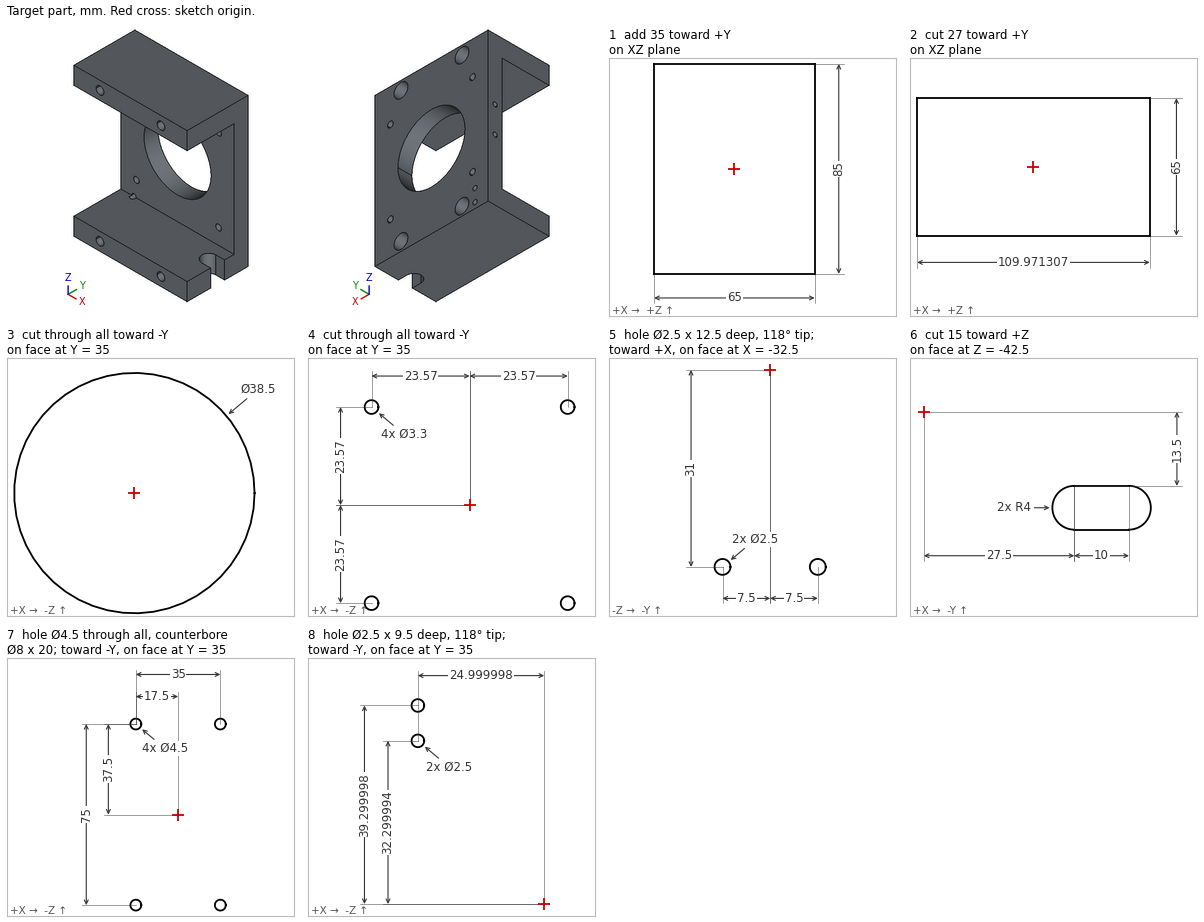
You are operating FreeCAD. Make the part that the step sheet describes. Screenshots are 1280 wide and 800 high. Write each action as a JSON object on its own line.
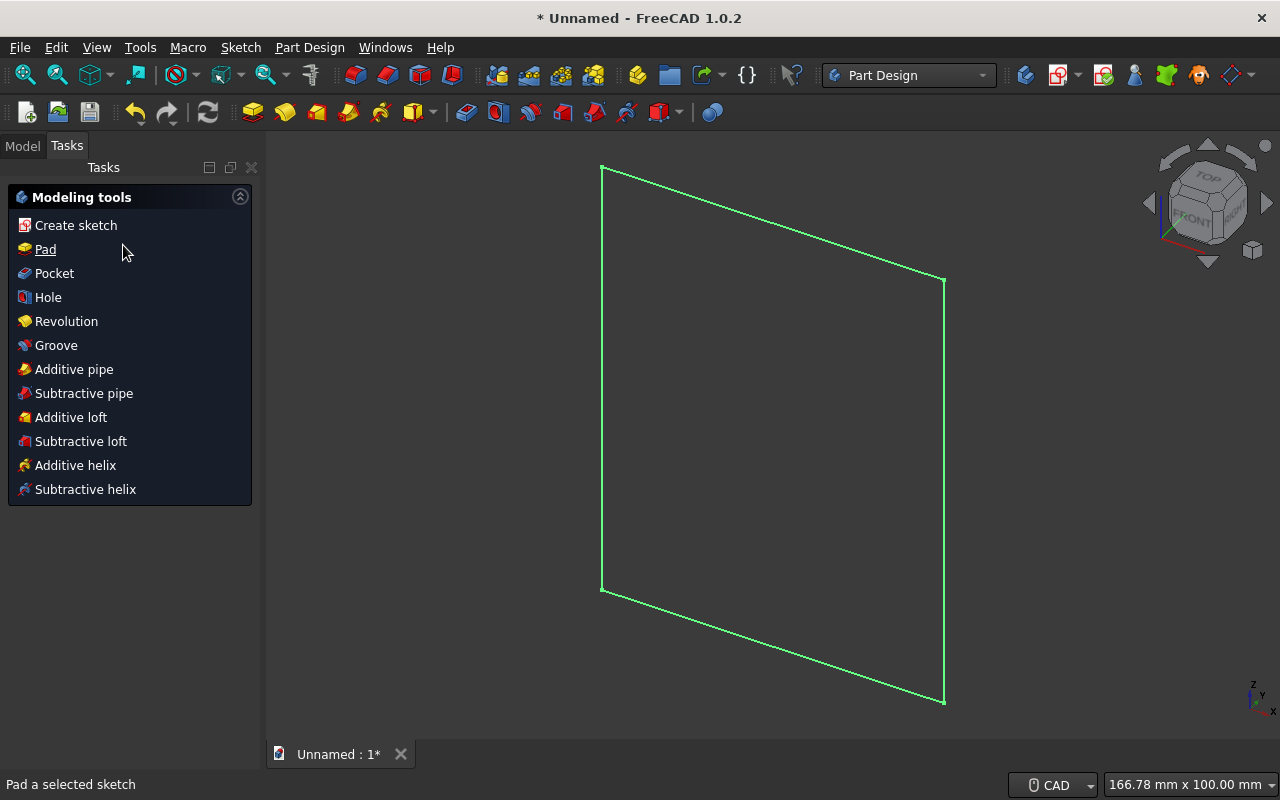
{"action": "left_click", "coordinate": [254, 112]}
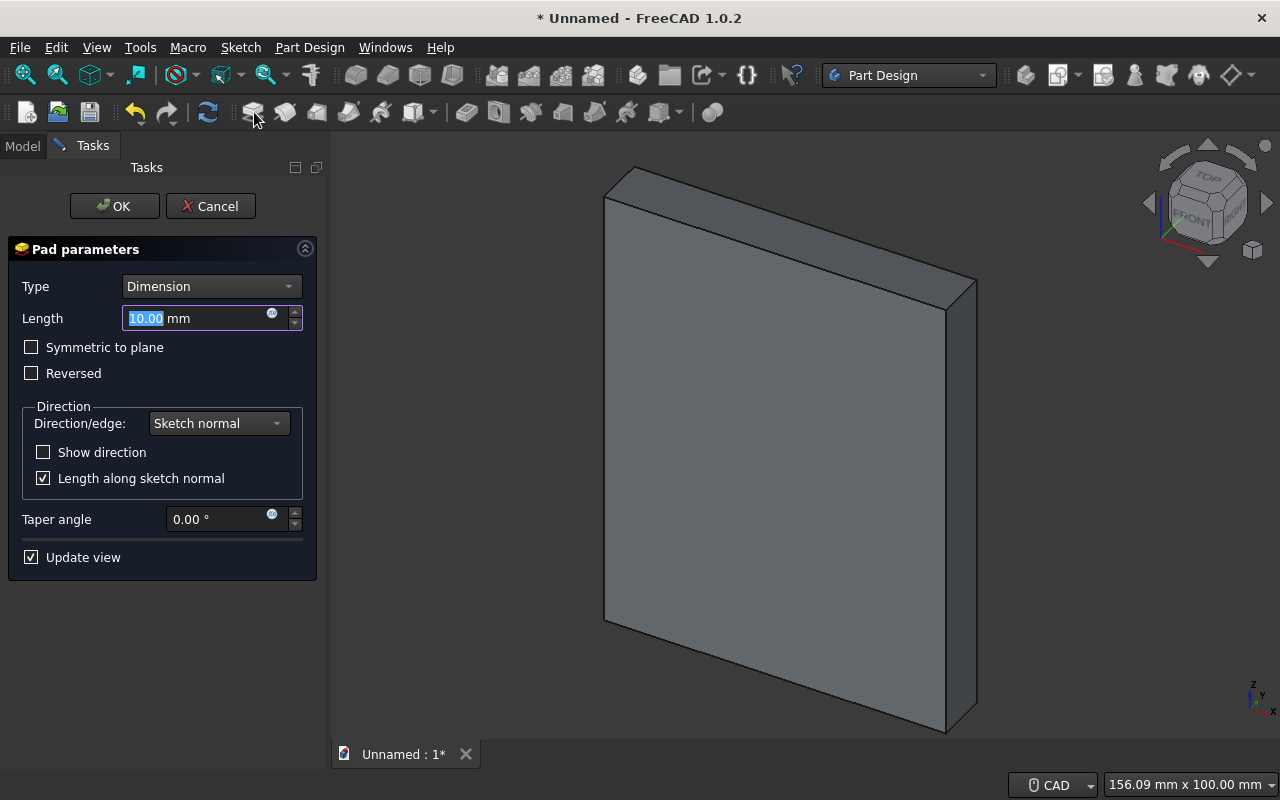
{"action": "type", "text": "35"}
{"action": "key", "text": "Tab"}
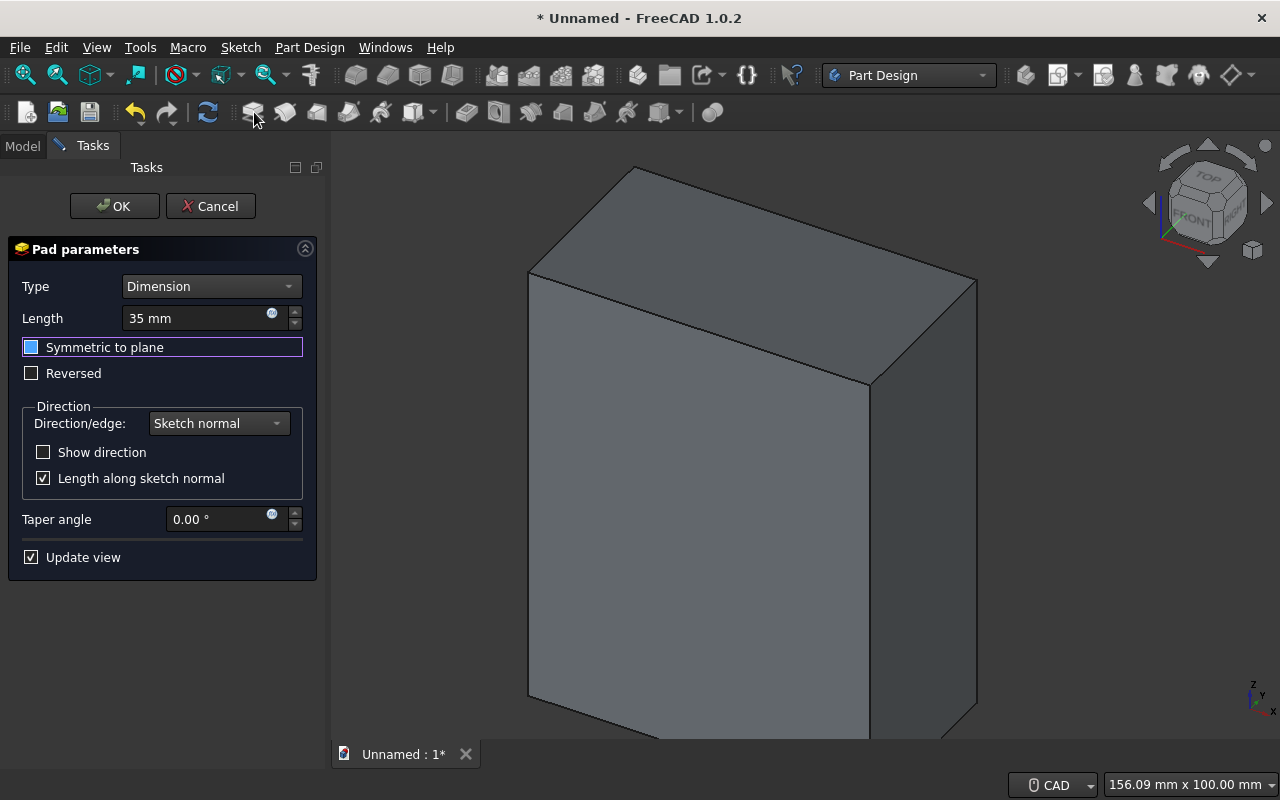
{"action": "left_click", "coordinate": [30, 373]}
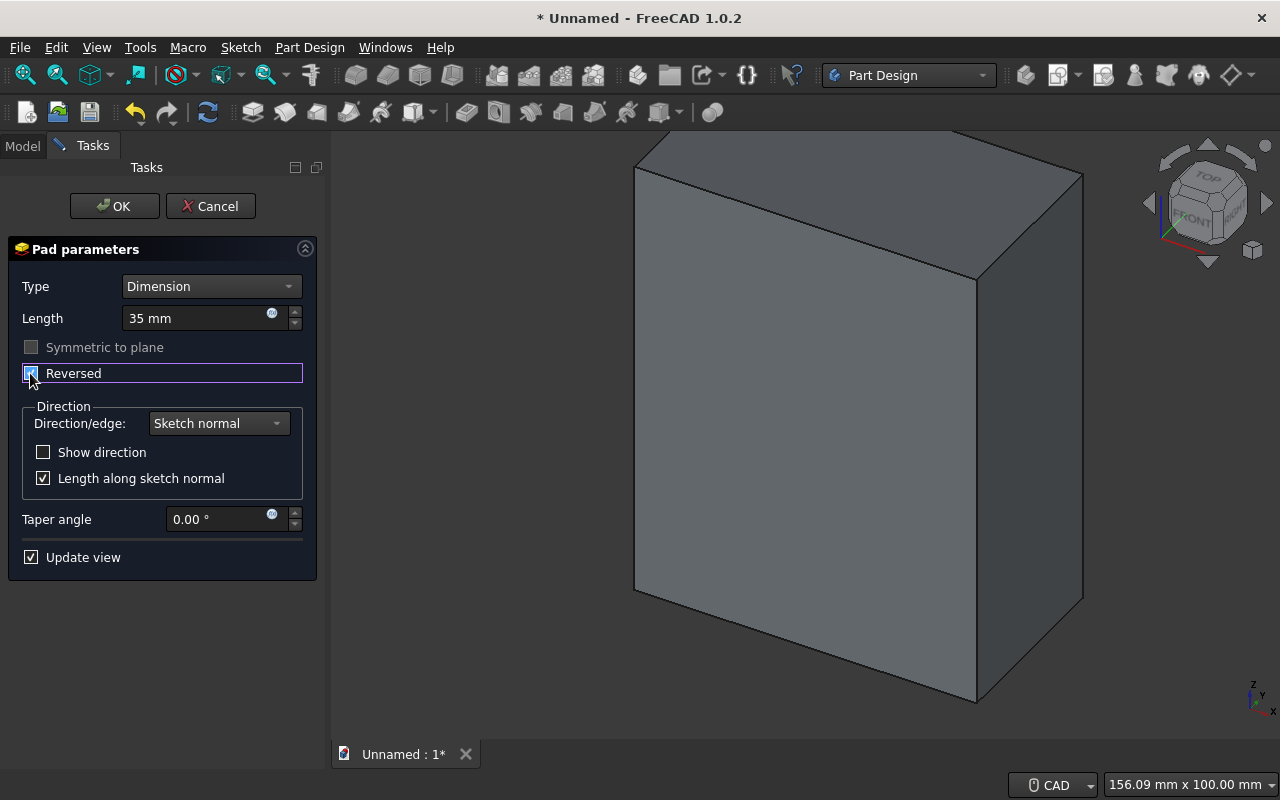
{"action": "left_click", "coordinate": [115, 206]}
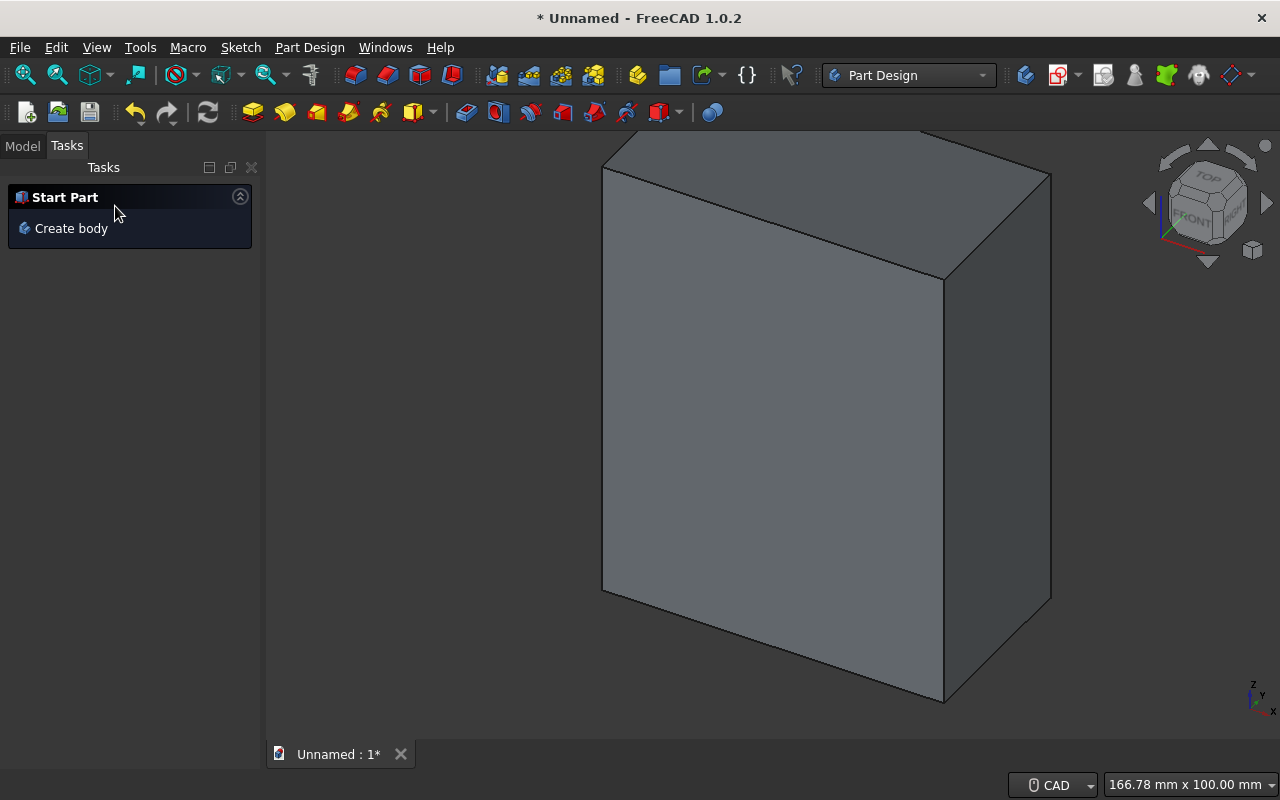
{"action": "left_click", "coordinate": [26, 76]}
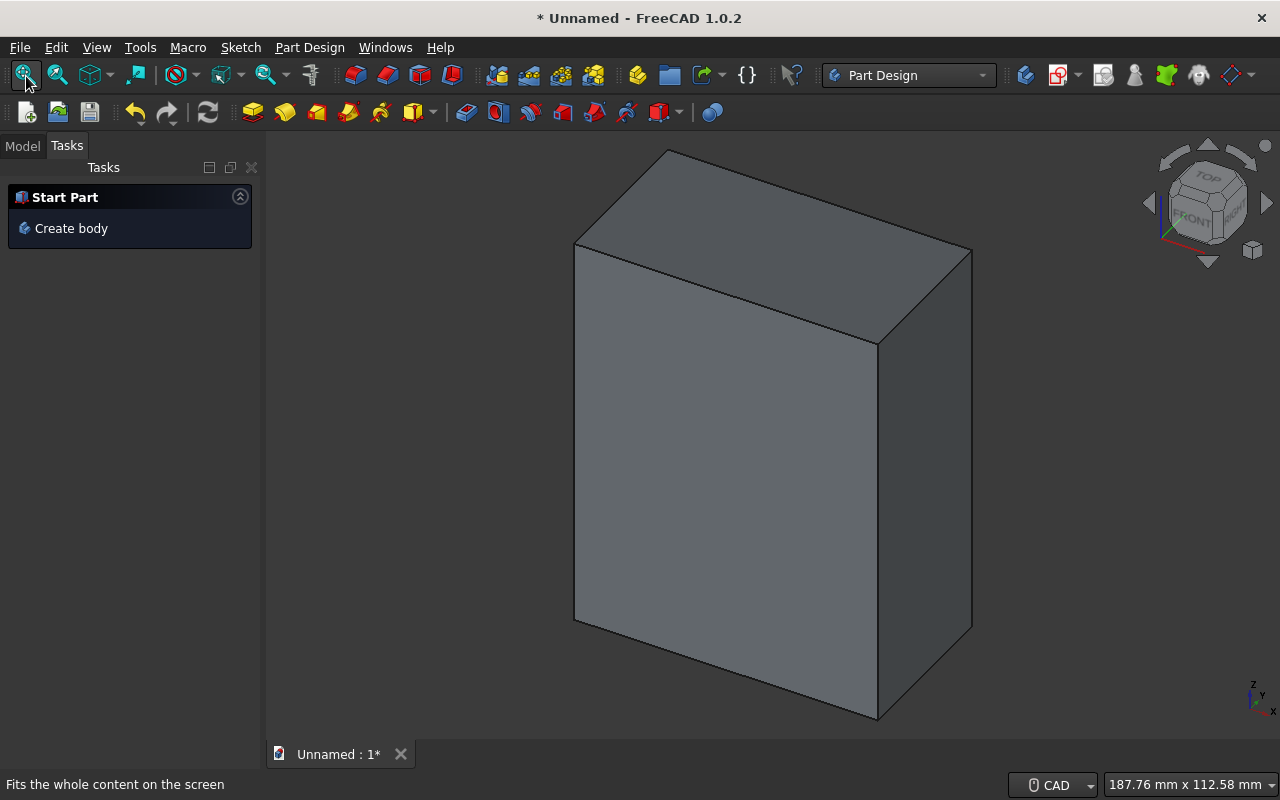
{"action": "left_click", "coordinate": [1058, 76]}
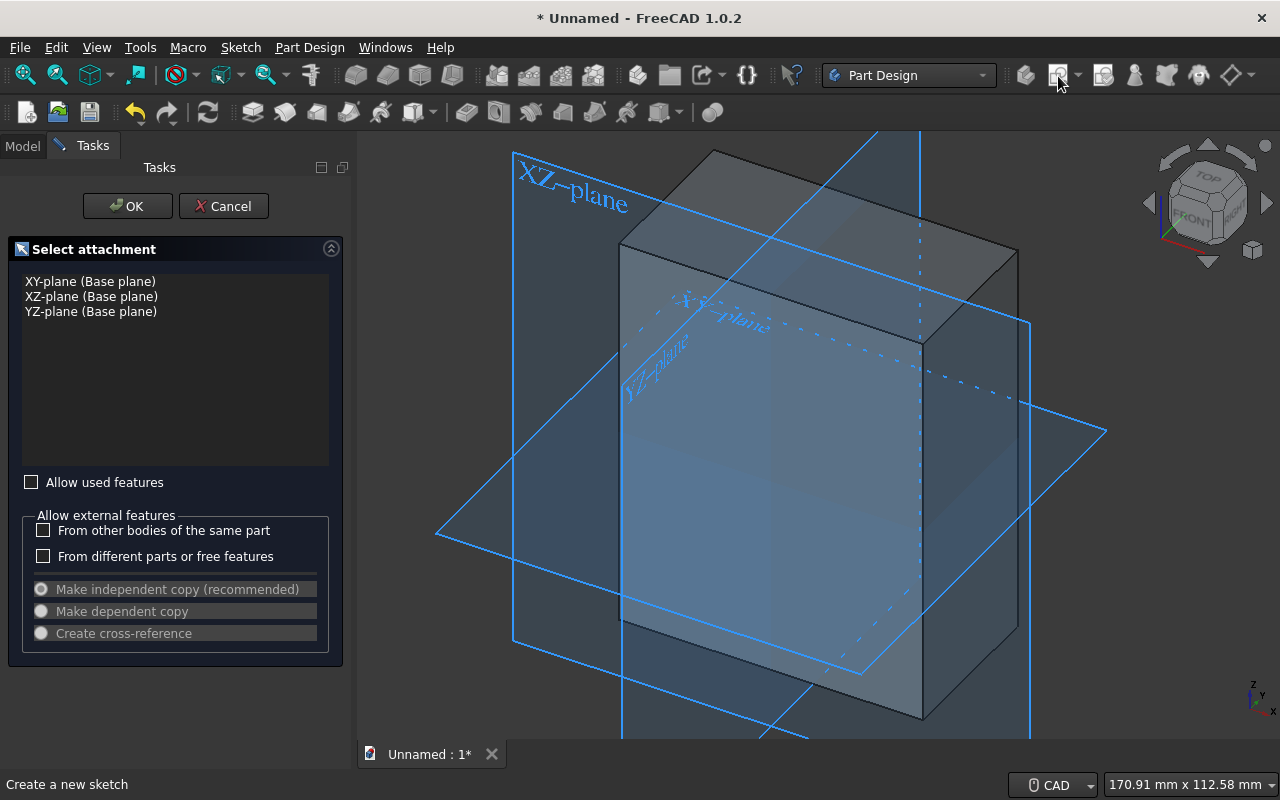
{"action": "left_click", "coordinate": [82, 296]}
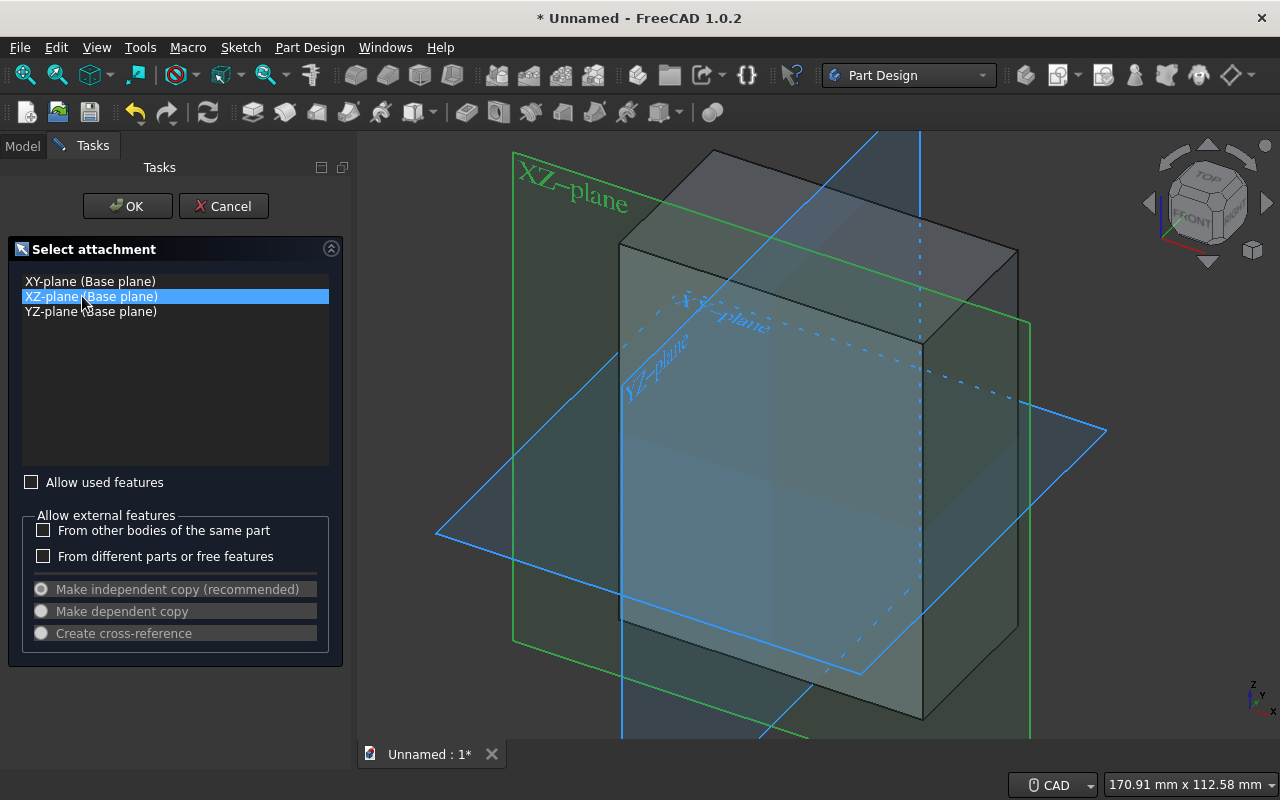
{"action": "left_click", "coordinate": [128, 206]}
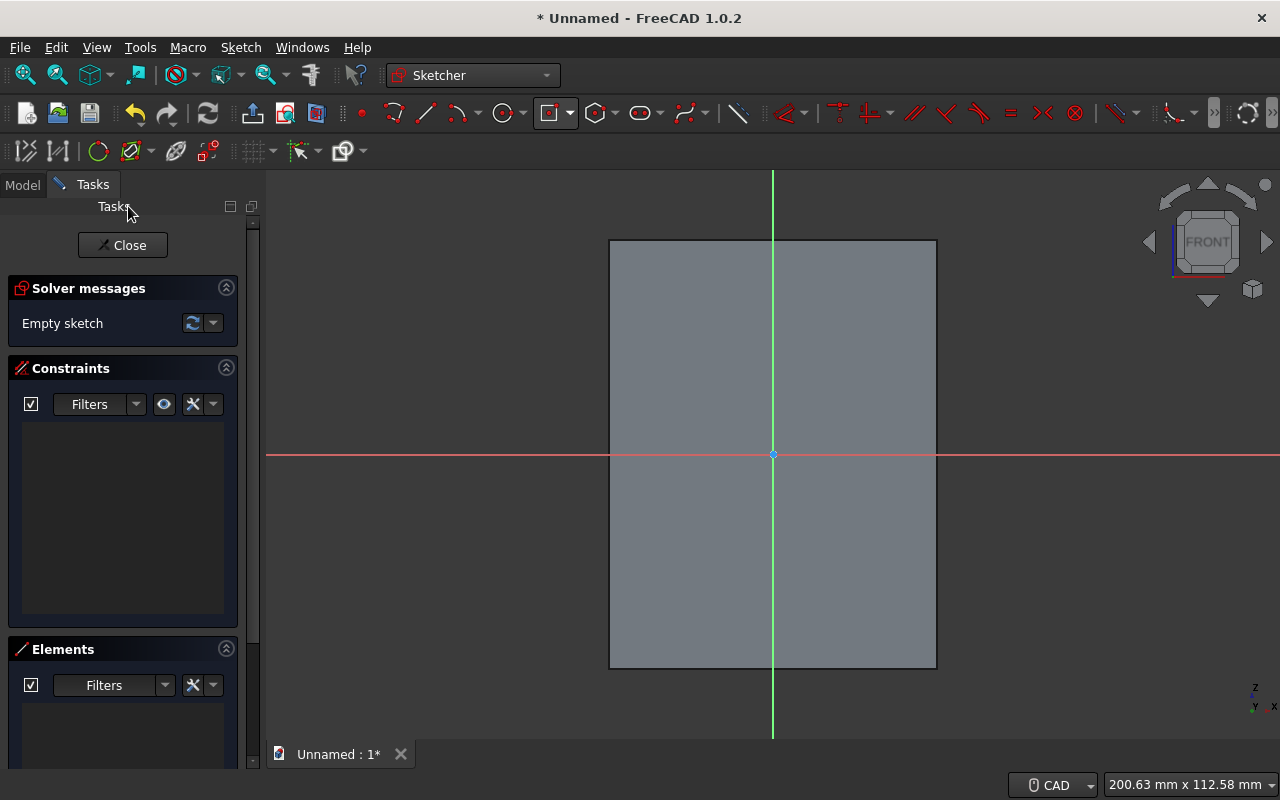
{"action": "left_click", "coordinate": [550, 114]}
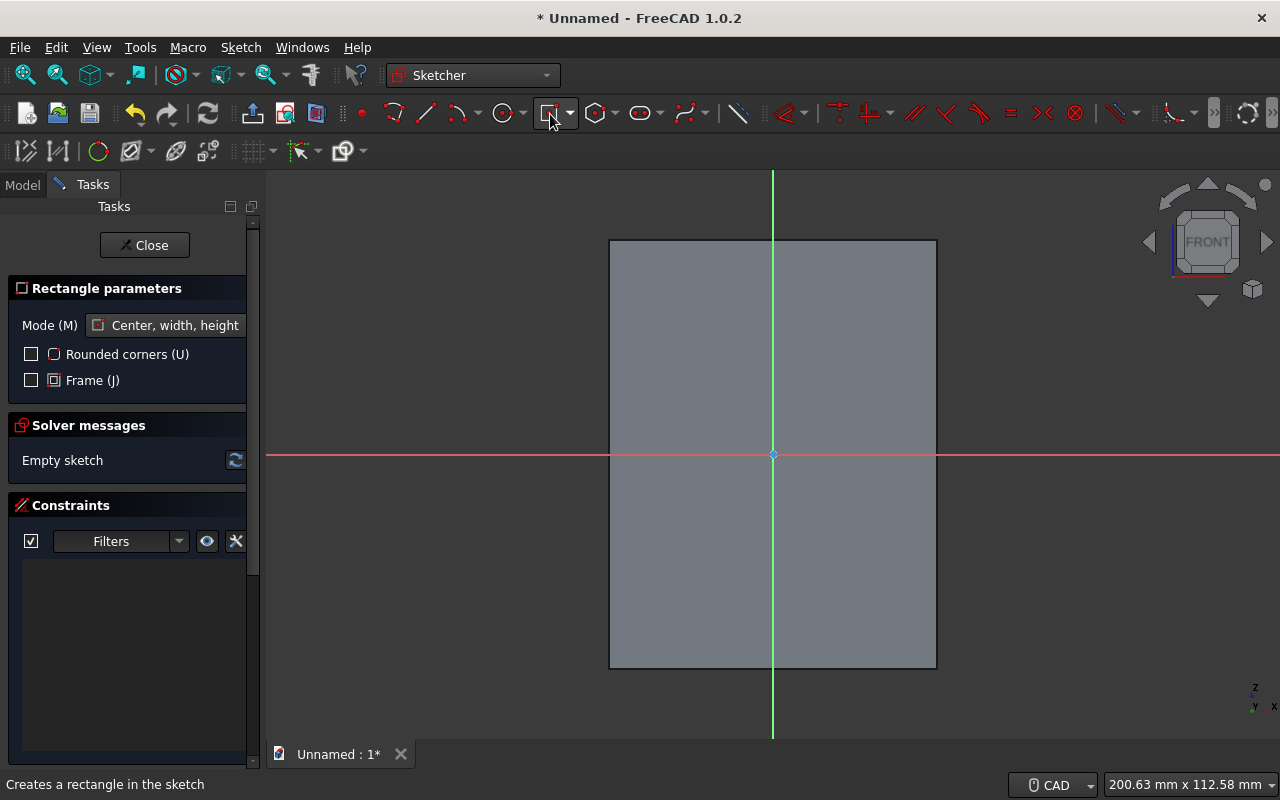
{"action": "left_click", "coordinate": [773, 454]}
{"action": "mouse_move", "coordinate": [1051, 290]}